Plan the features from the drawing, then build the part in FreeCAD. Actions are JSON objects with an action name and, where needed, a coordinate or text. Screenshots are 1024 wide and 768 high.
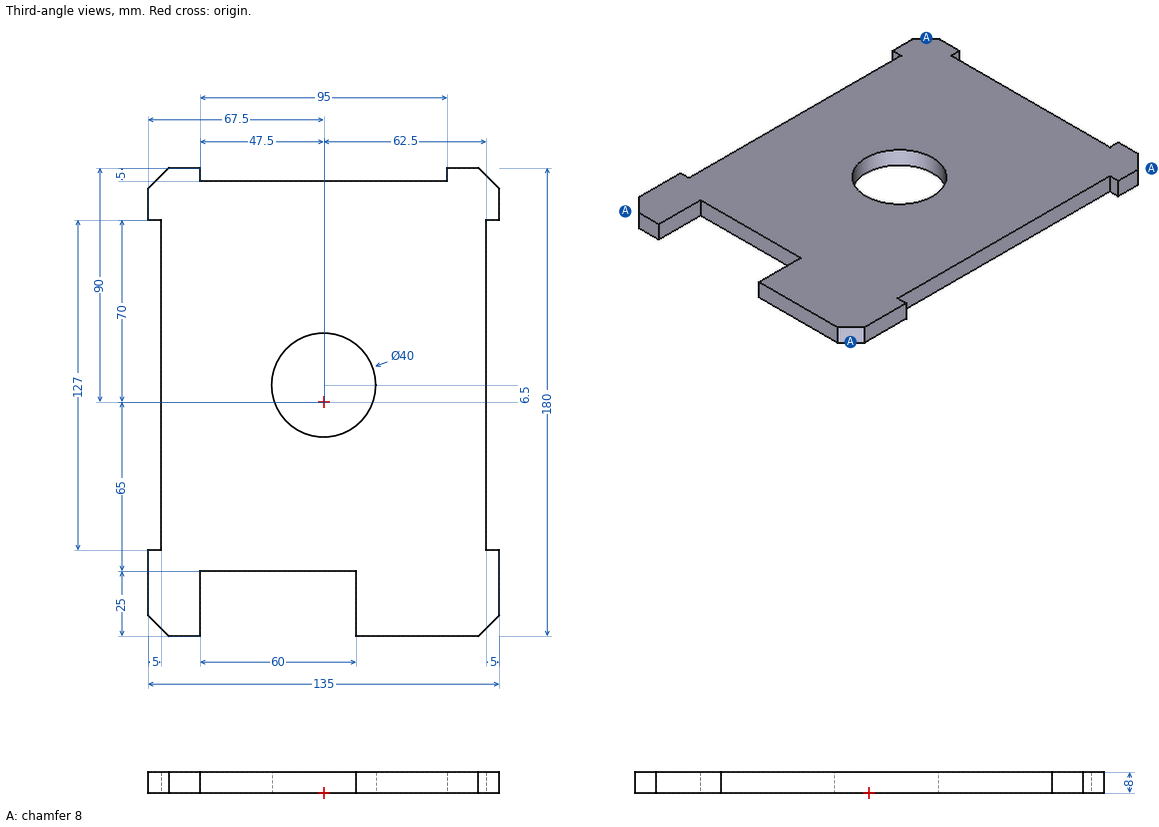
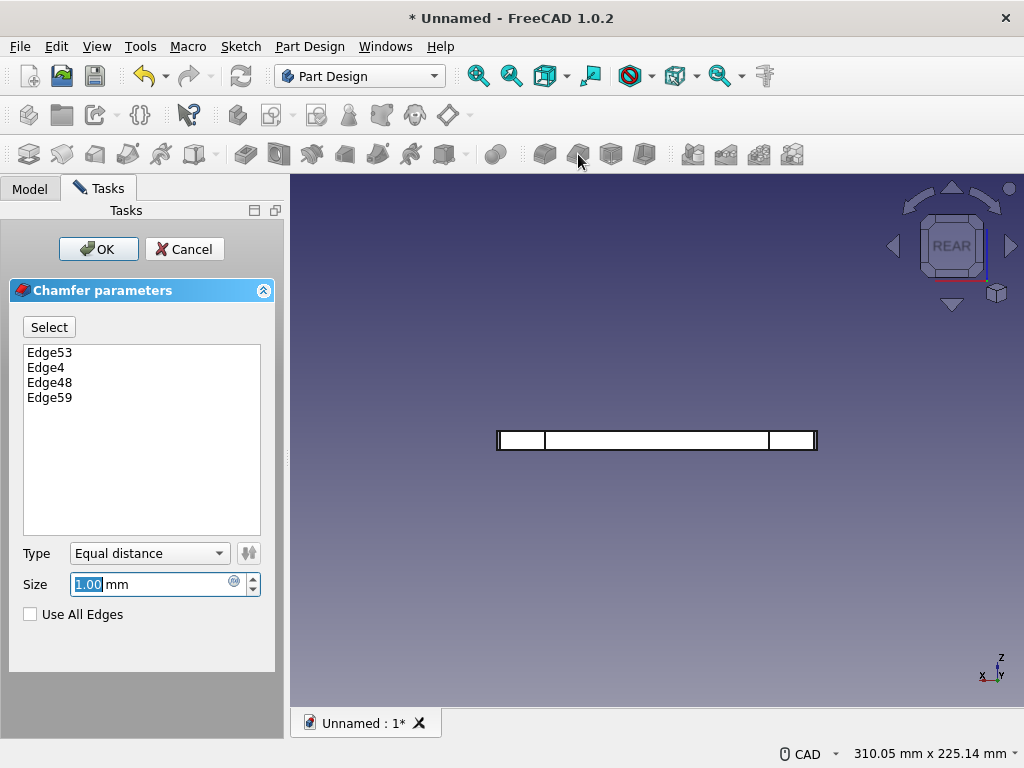
{"action": "type", "text": "8"}
{"action": "key", "text": "Tab"}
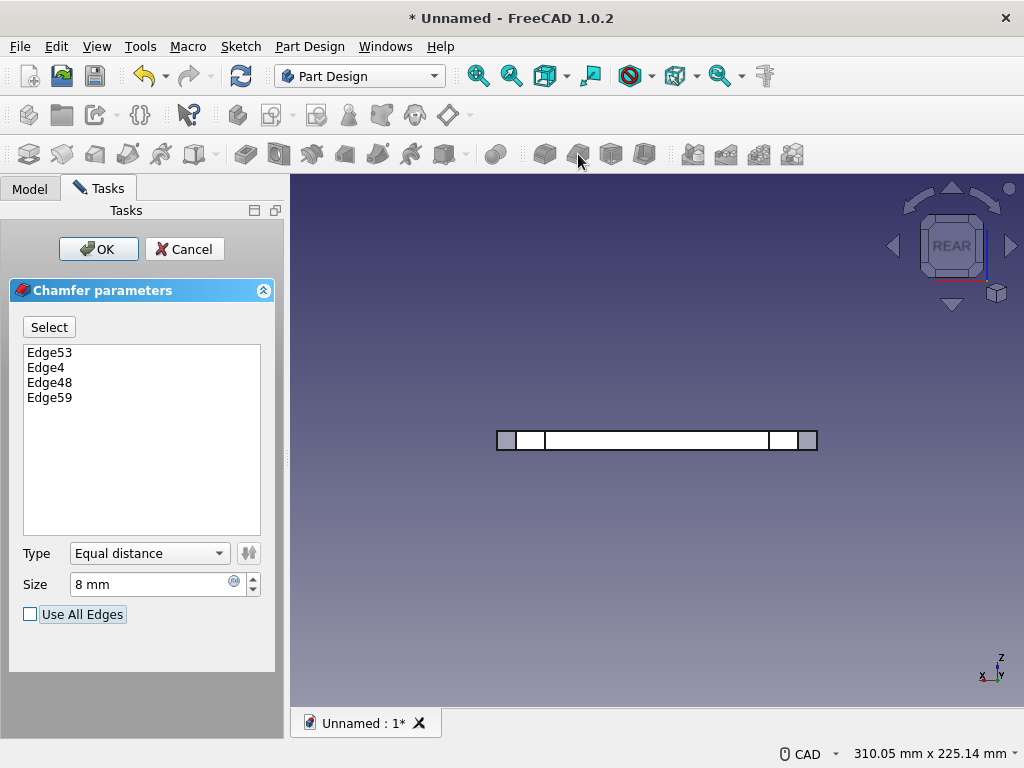
{"action": "left_click", "coordinate": [99, 249]}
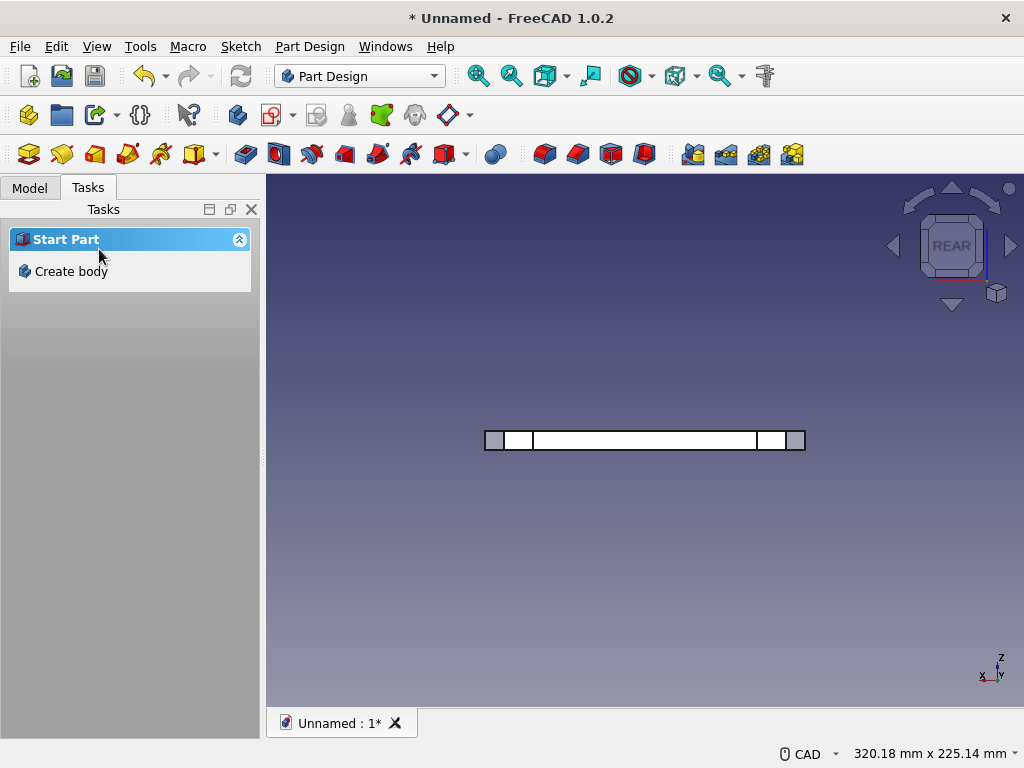
{"action": "key", "text": "v f"}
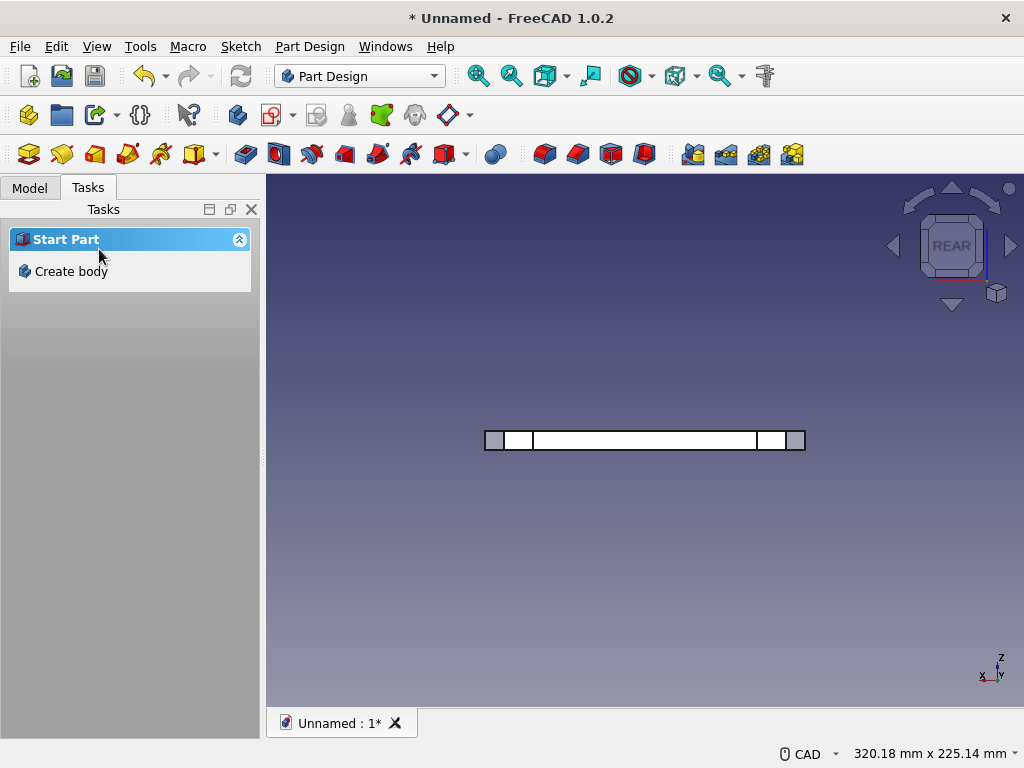
{"action": "key", "text": "0"}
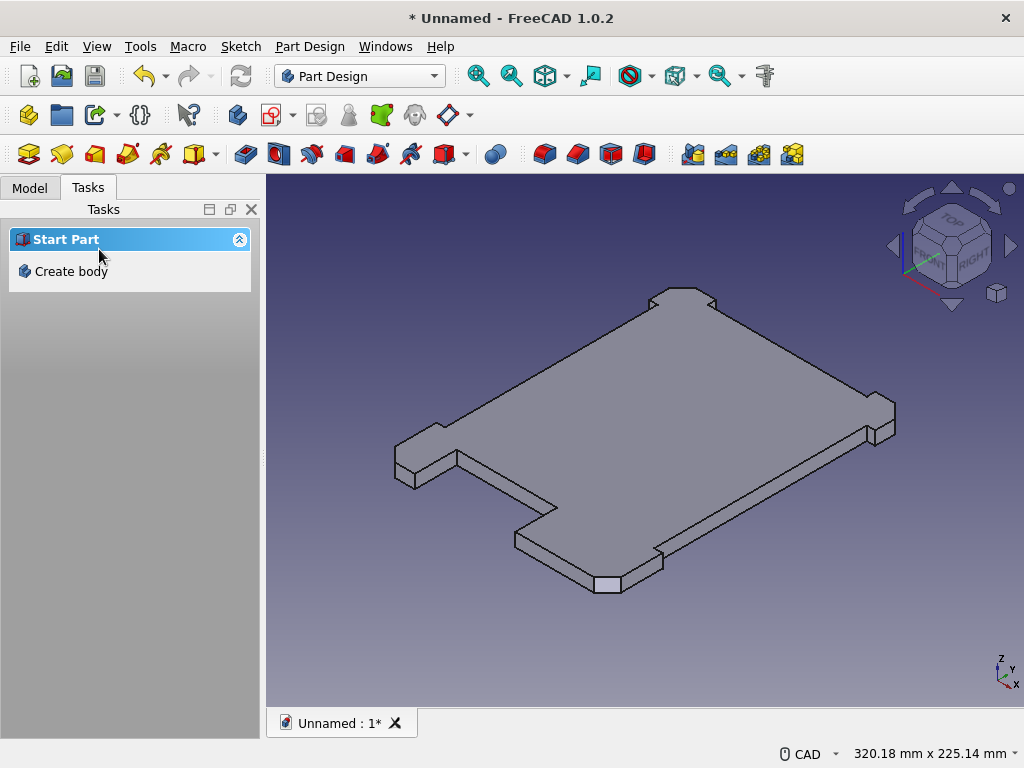
{"action": "left_click", "coordinate": [645, 432]}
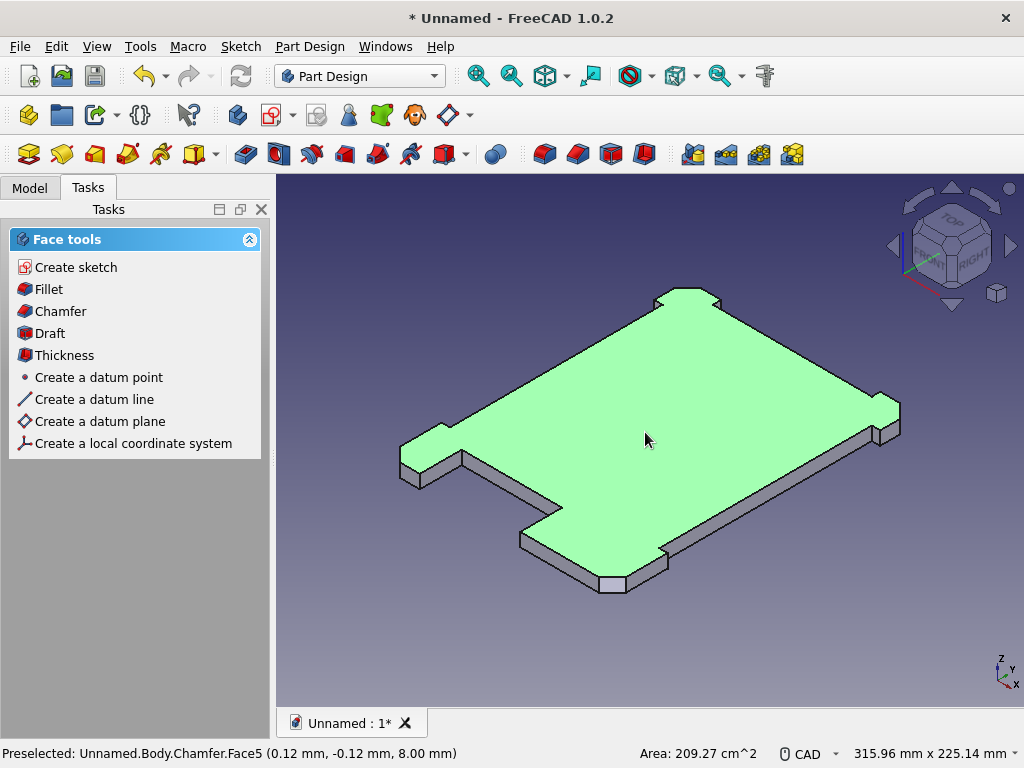
{"action": "left_click", "coordinate": [270, 116]}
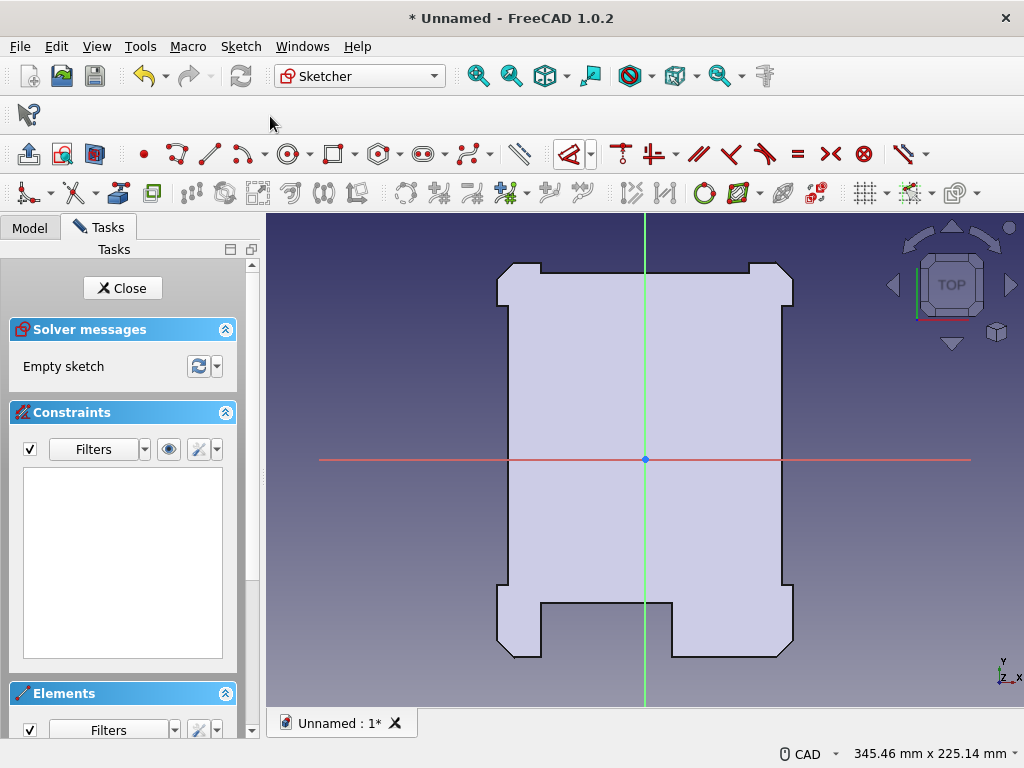
{"action": "scroll", "coordinate": [675, 440], "scroll_direction": "up", "scroll_amount": 6}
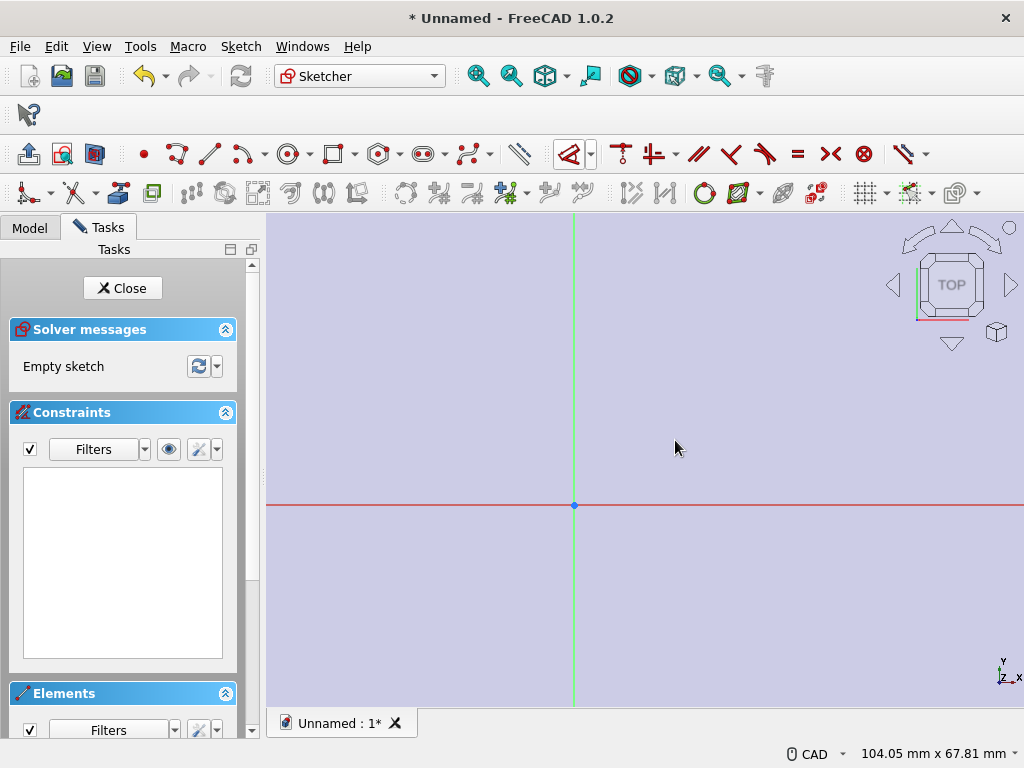
{"action": "key", "text": "g c"}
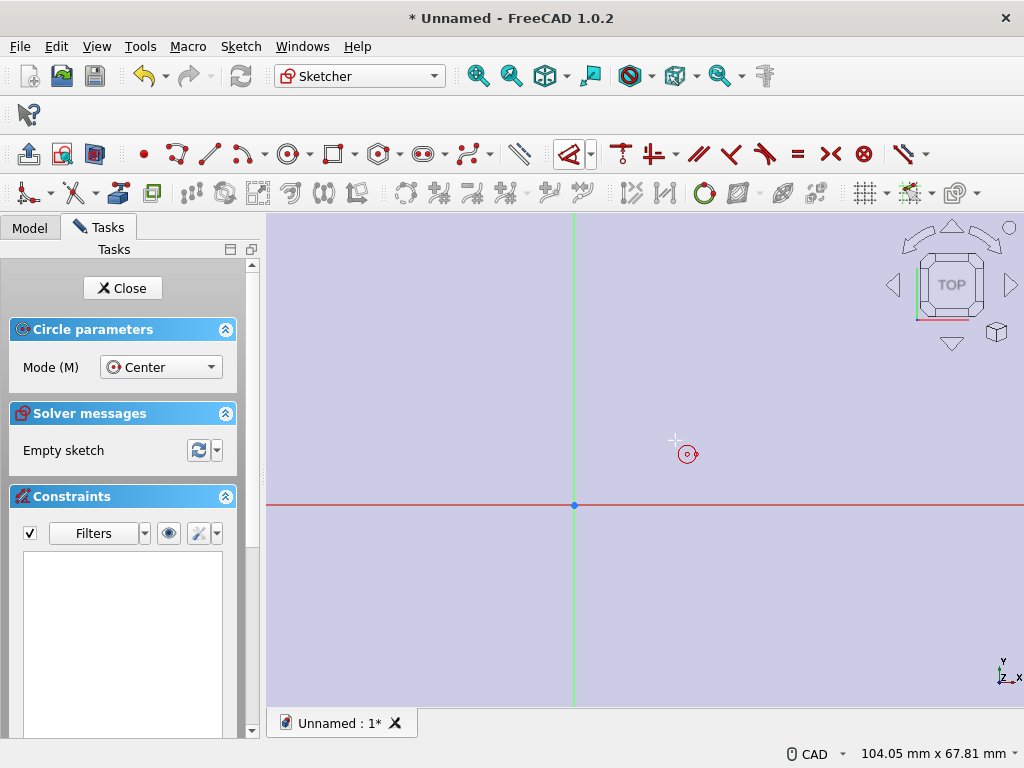
{"action": "left_click", "coordinate": [574, 458]}
{"action": "left_click", "coordinate": [677, 355]}
{"action": "key", "text": "Escape"}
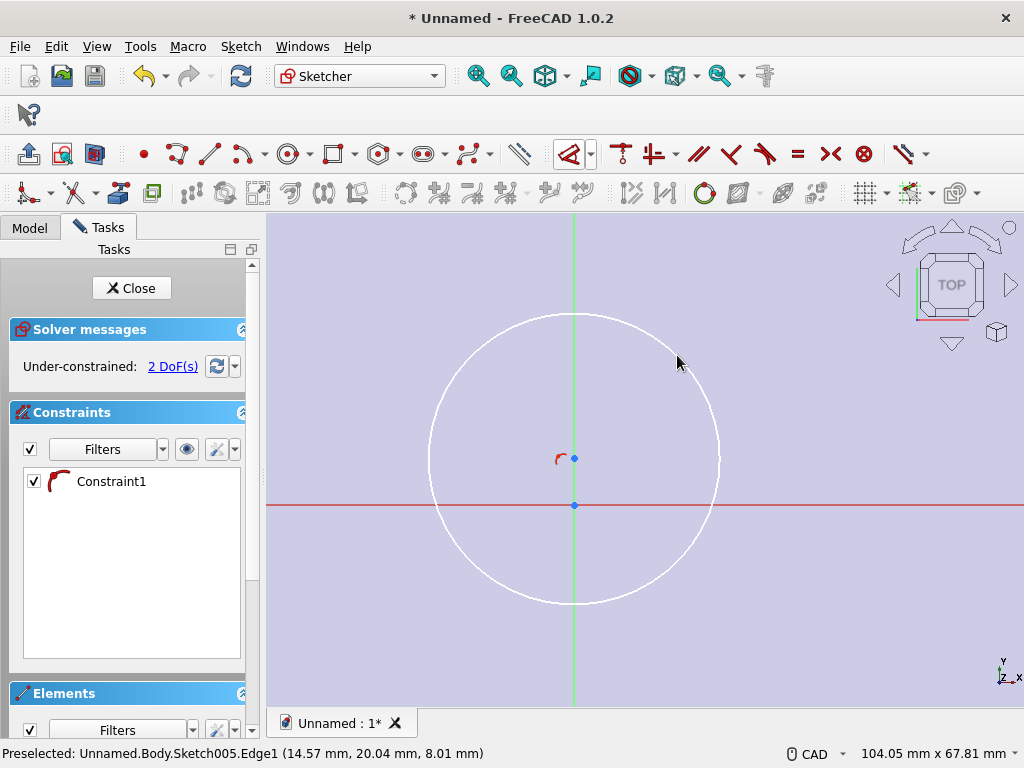
{"action": "left_click", "coordinate": [677, 356]}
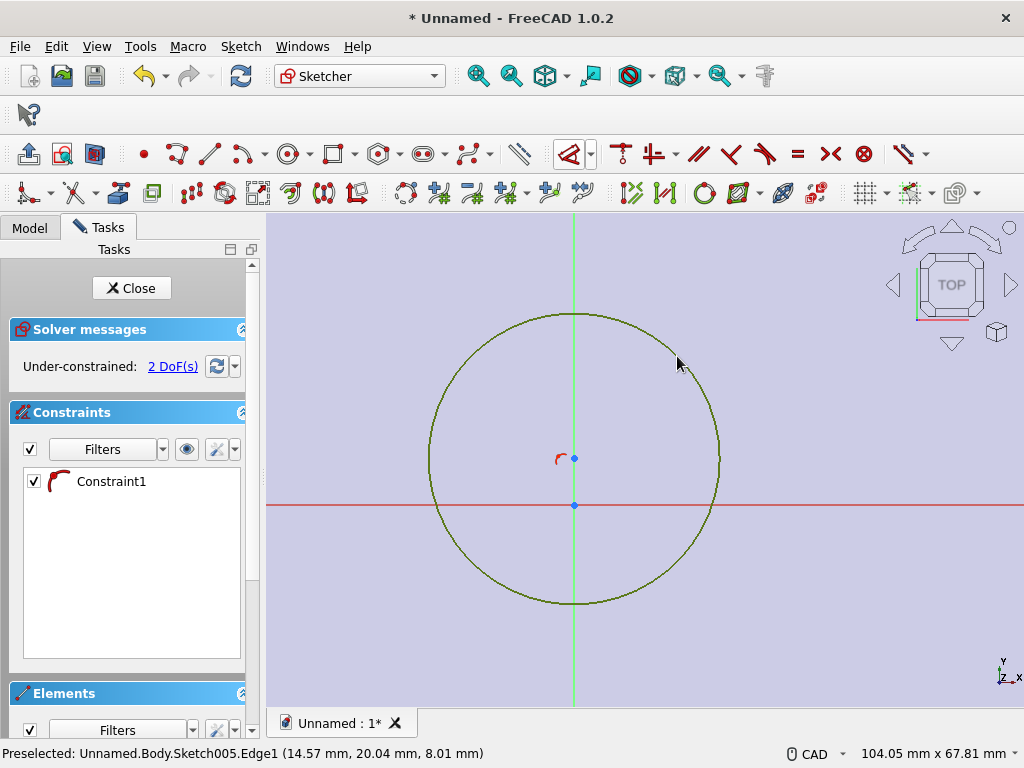
{"action": "key", "text": "k o"}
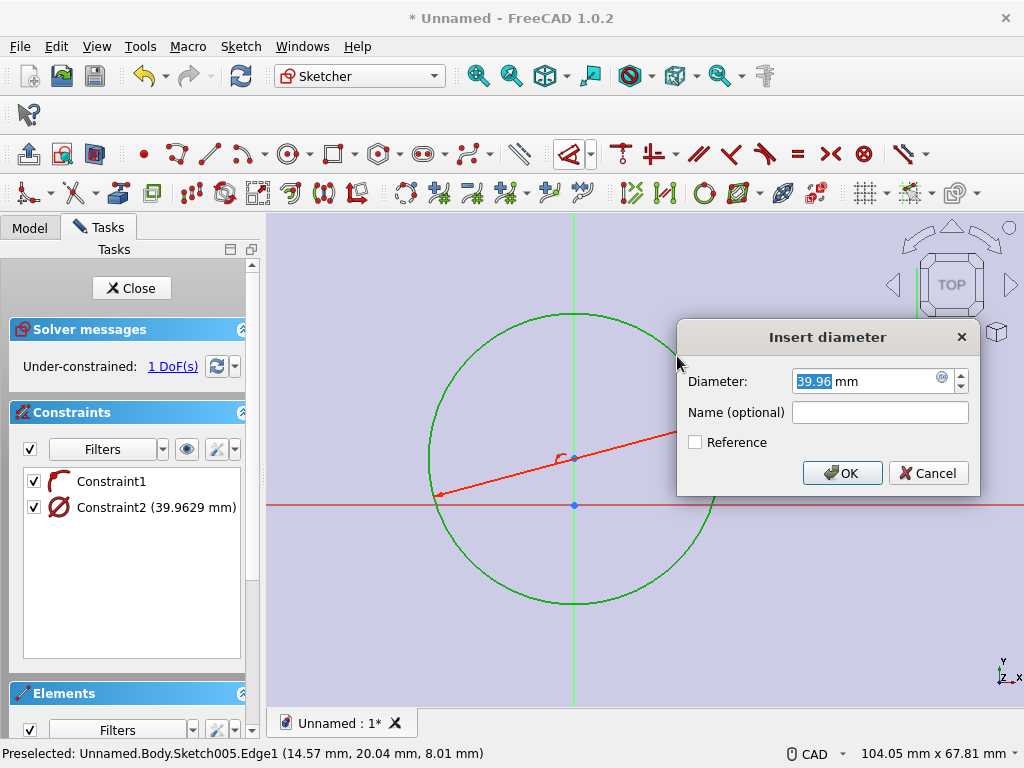
{"action": "type", "text": "40"}
{"action": "key", "text": "Return"}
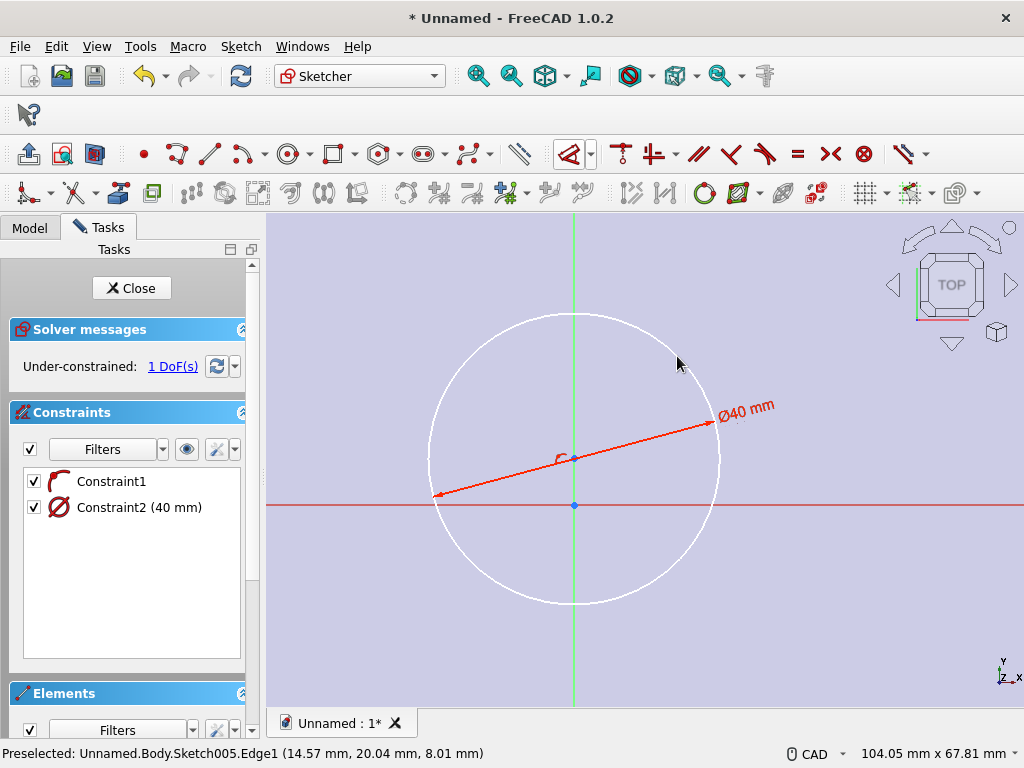
{"action": "left_click", "coordinate": [574, 459]}